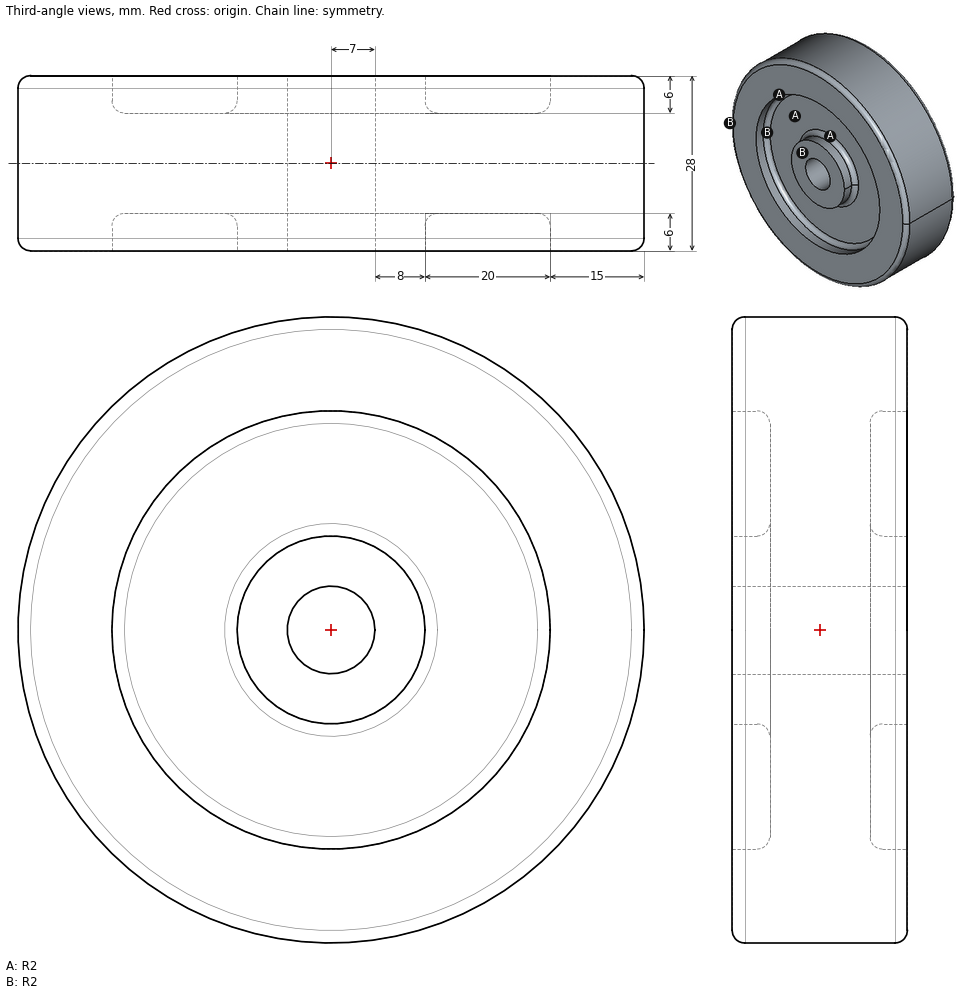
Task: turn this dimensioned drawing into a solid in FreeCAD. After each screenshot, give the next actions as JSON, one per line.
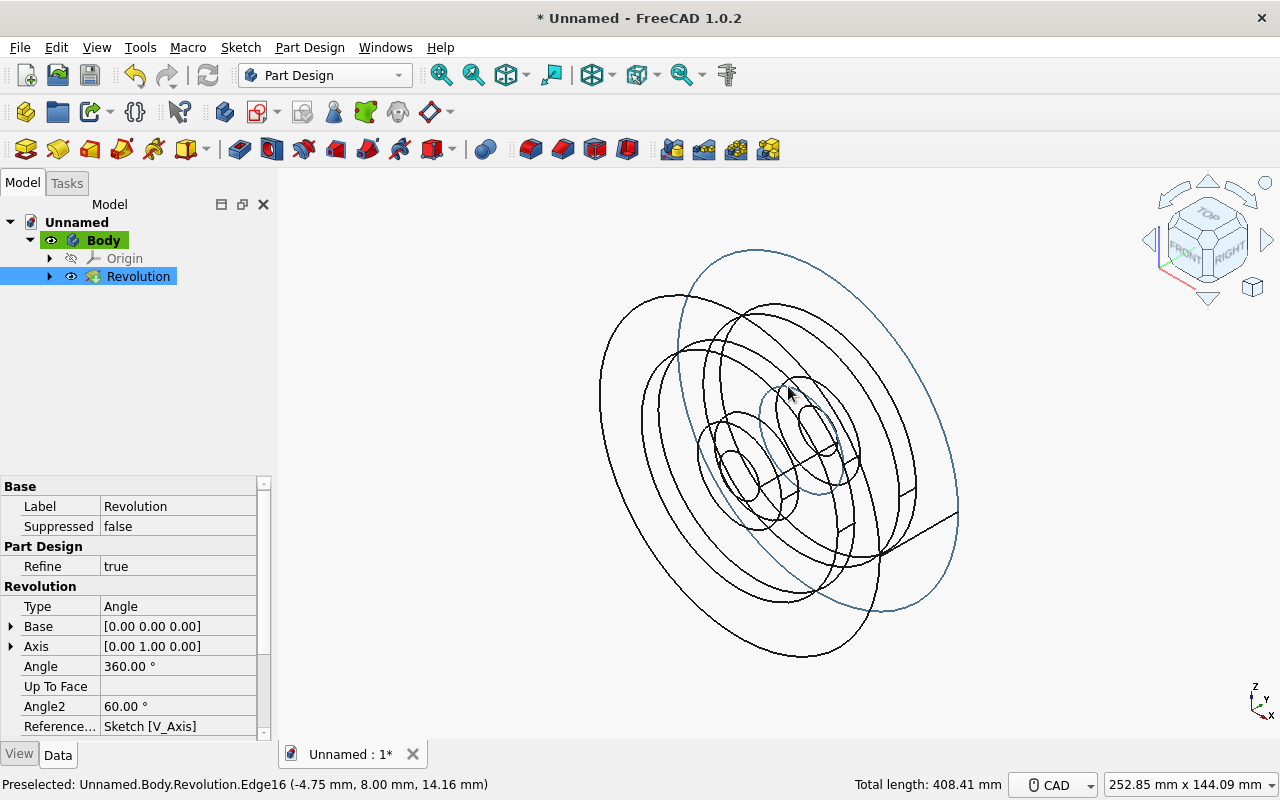
{"action": "left_click", "coordinate": [703, 383], "text": "ctrl"}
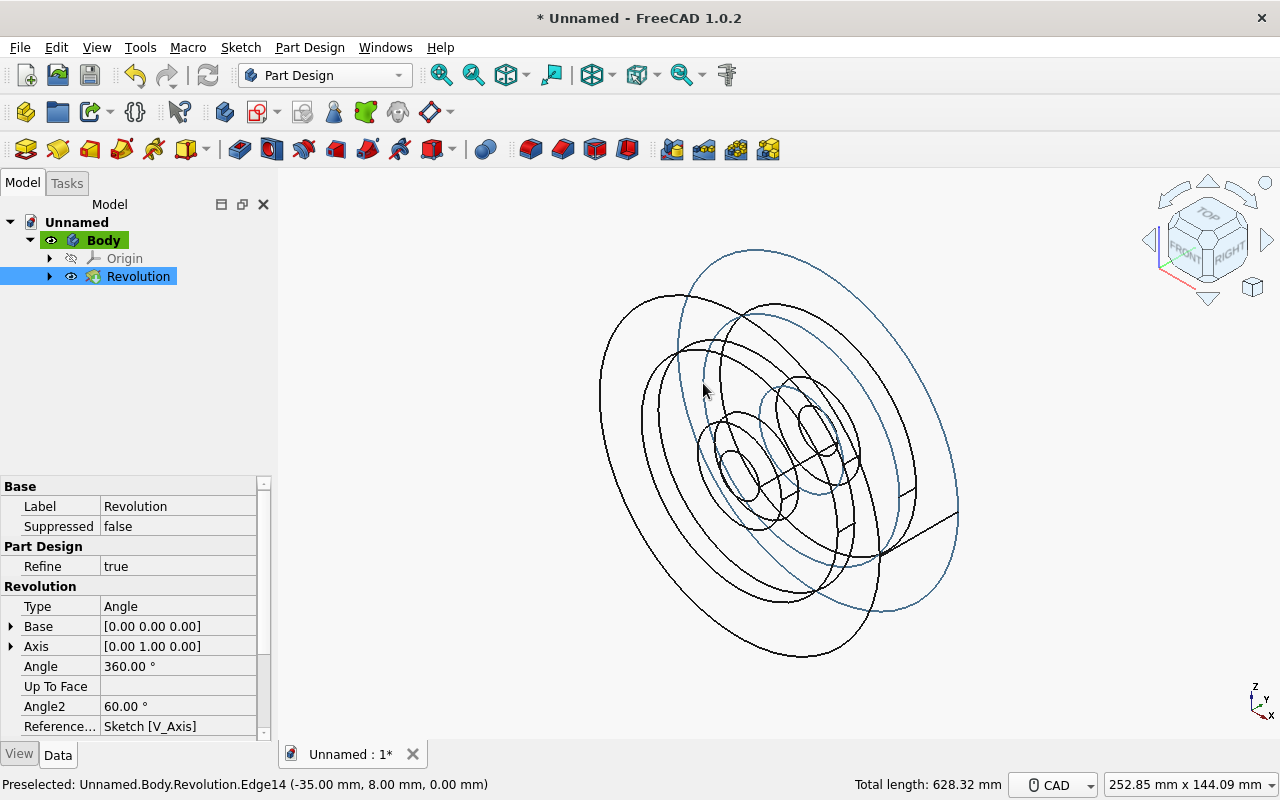
{"action": "key", "text": "v 1"}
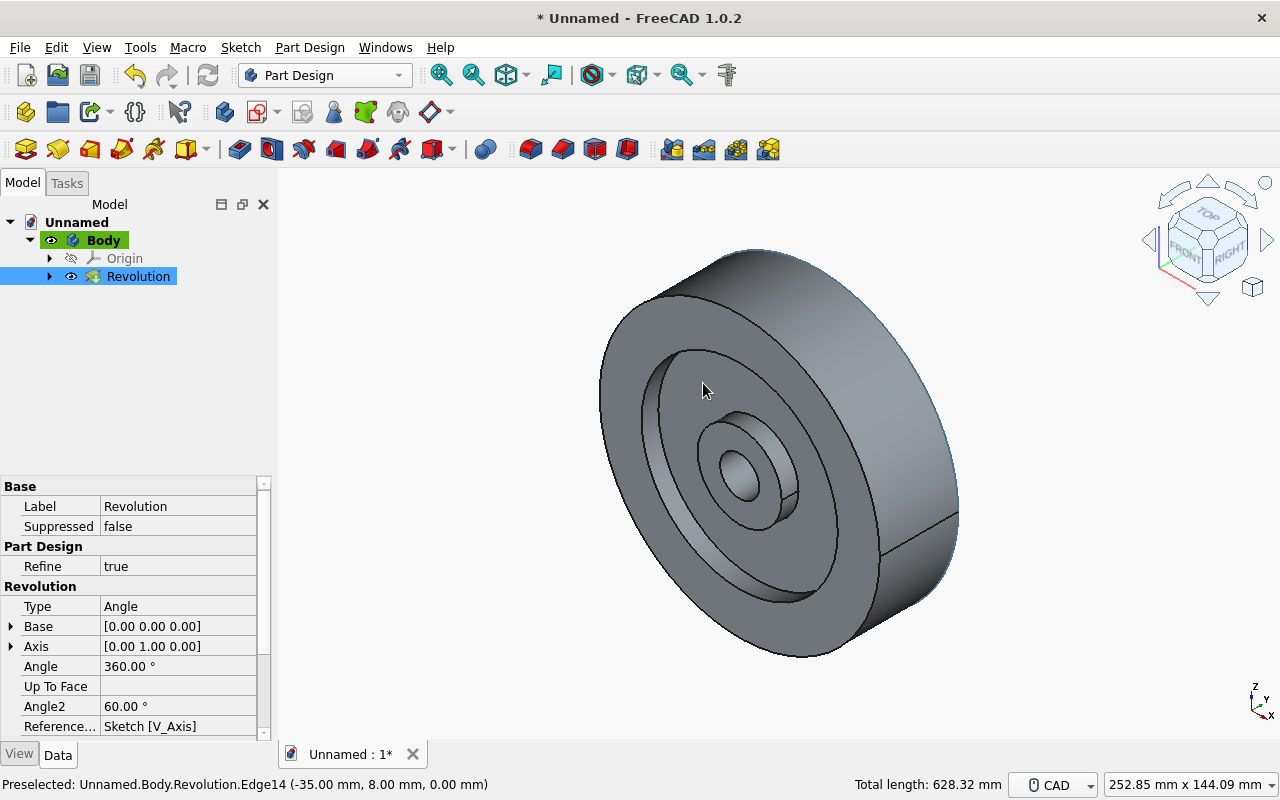
{"action": "left_click", "coordinate": [532, 150]}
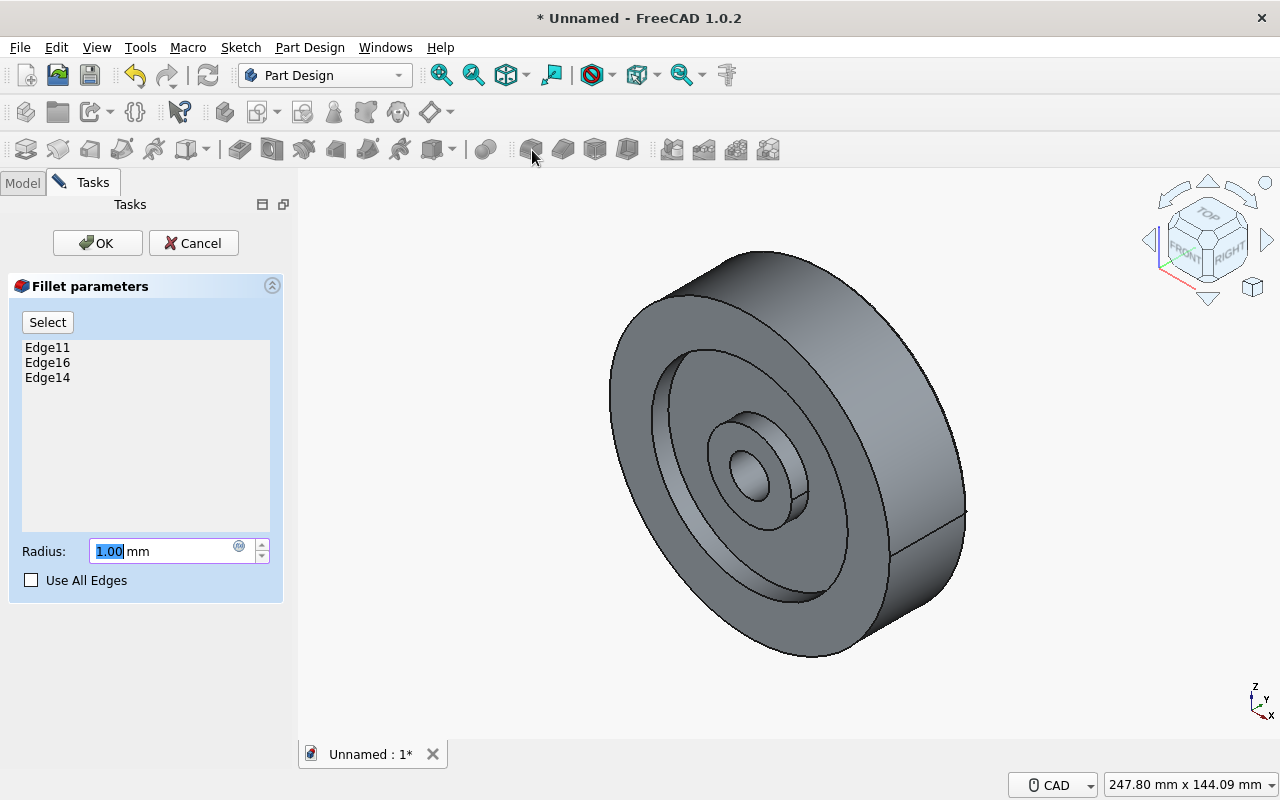
{"action": "type", "text": "2"}
{"action": "key", "text": "Tab"}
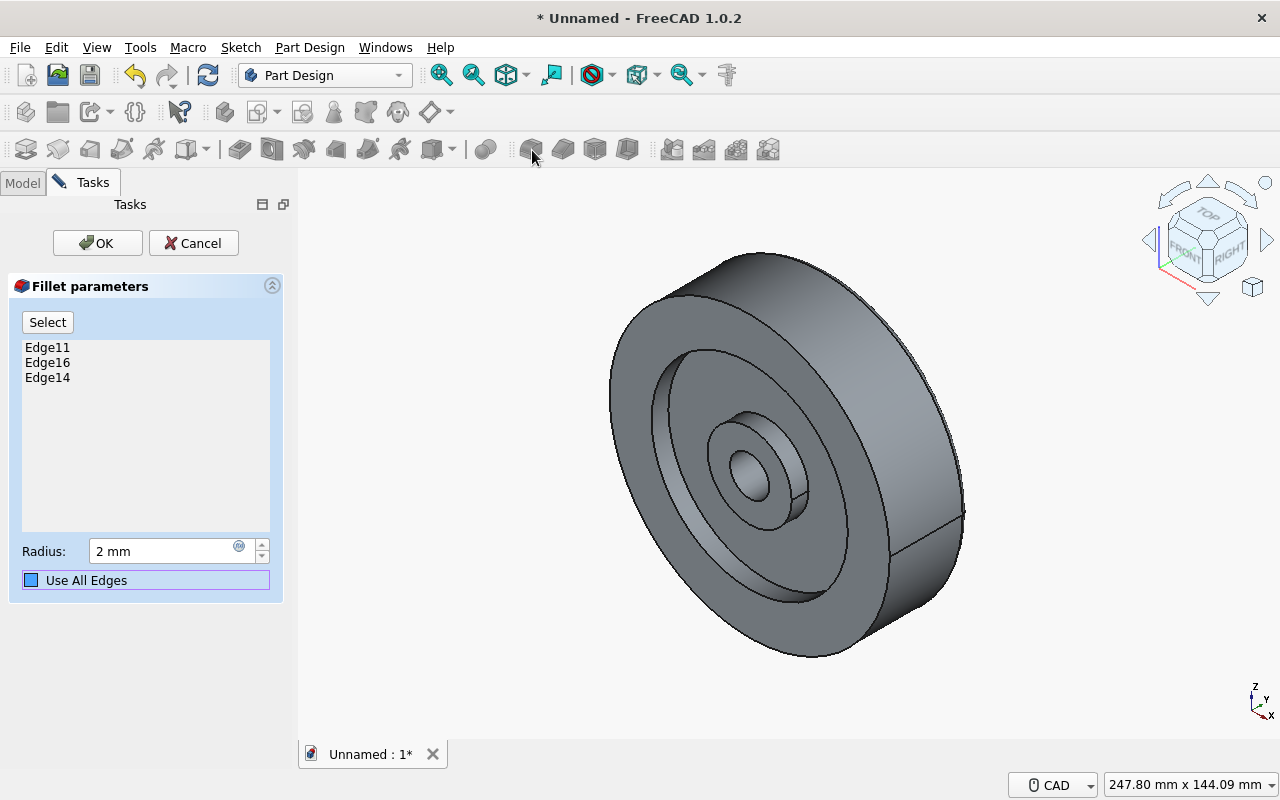
{"action": "left_click", "coordinate": [98, 243]}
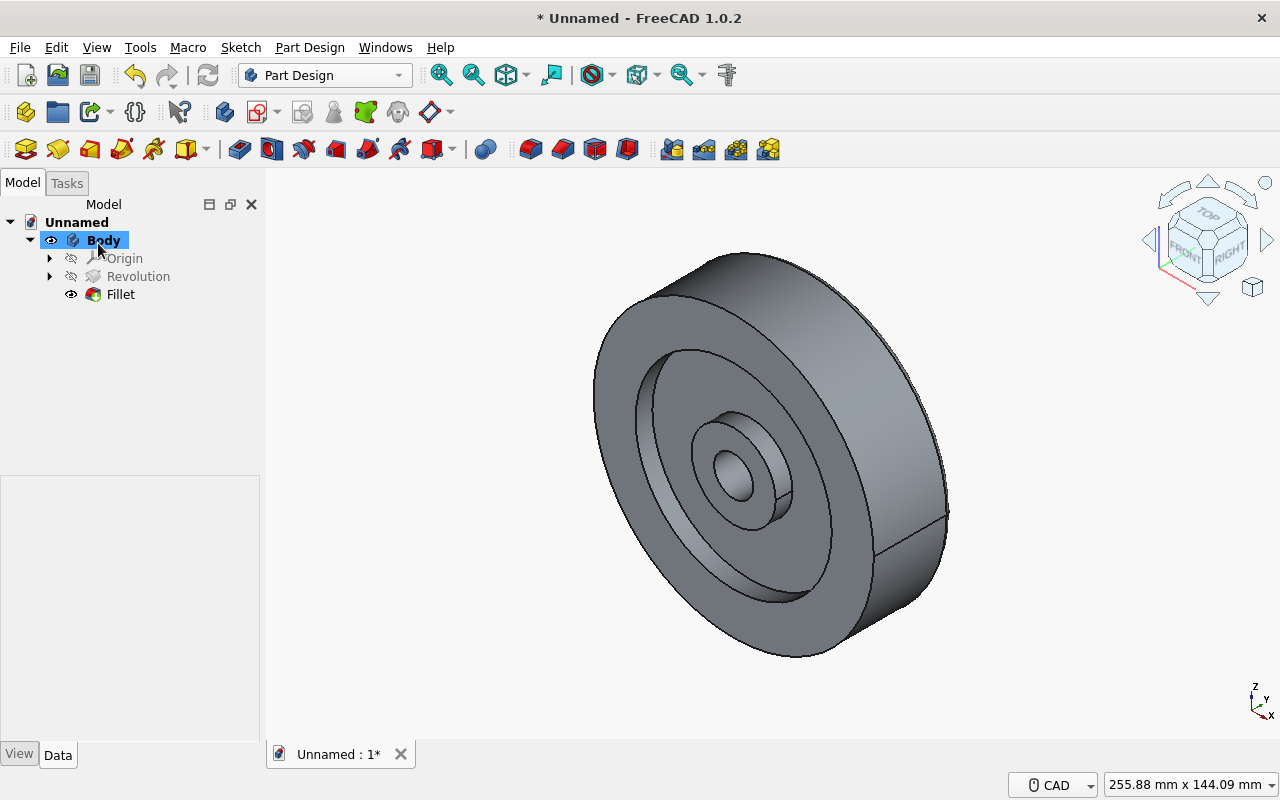
{"action": "left_click", "coordinate": [690, 296]}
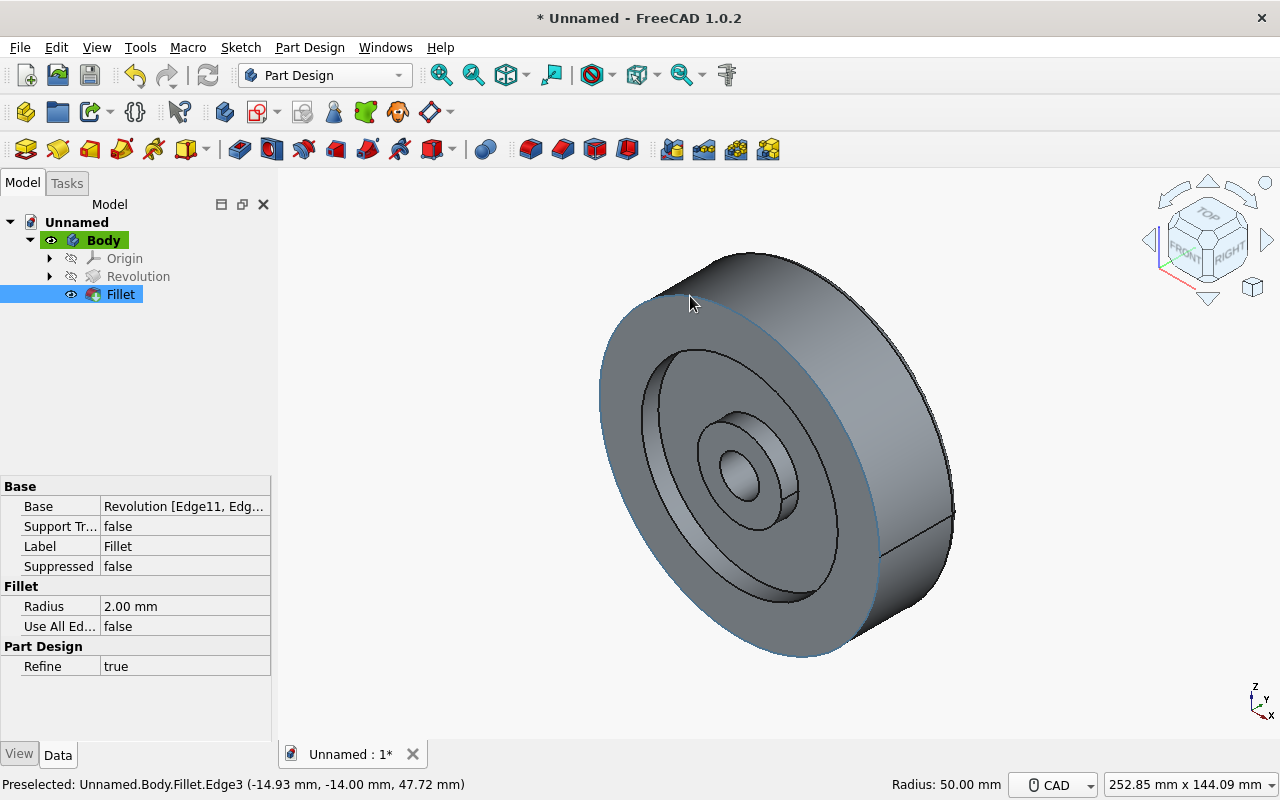
{"action": "key", "text": "2"}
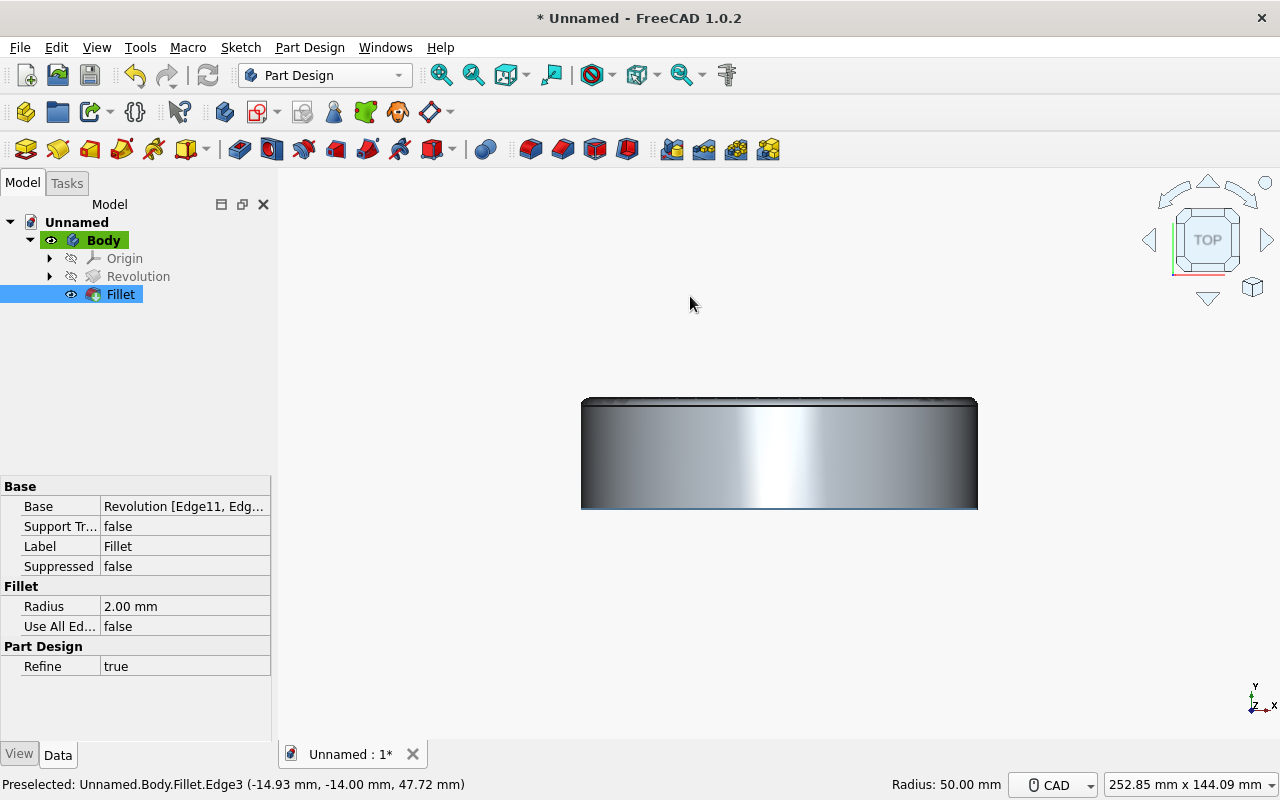
{"action": "left_click", "coordinate": [442, 76]}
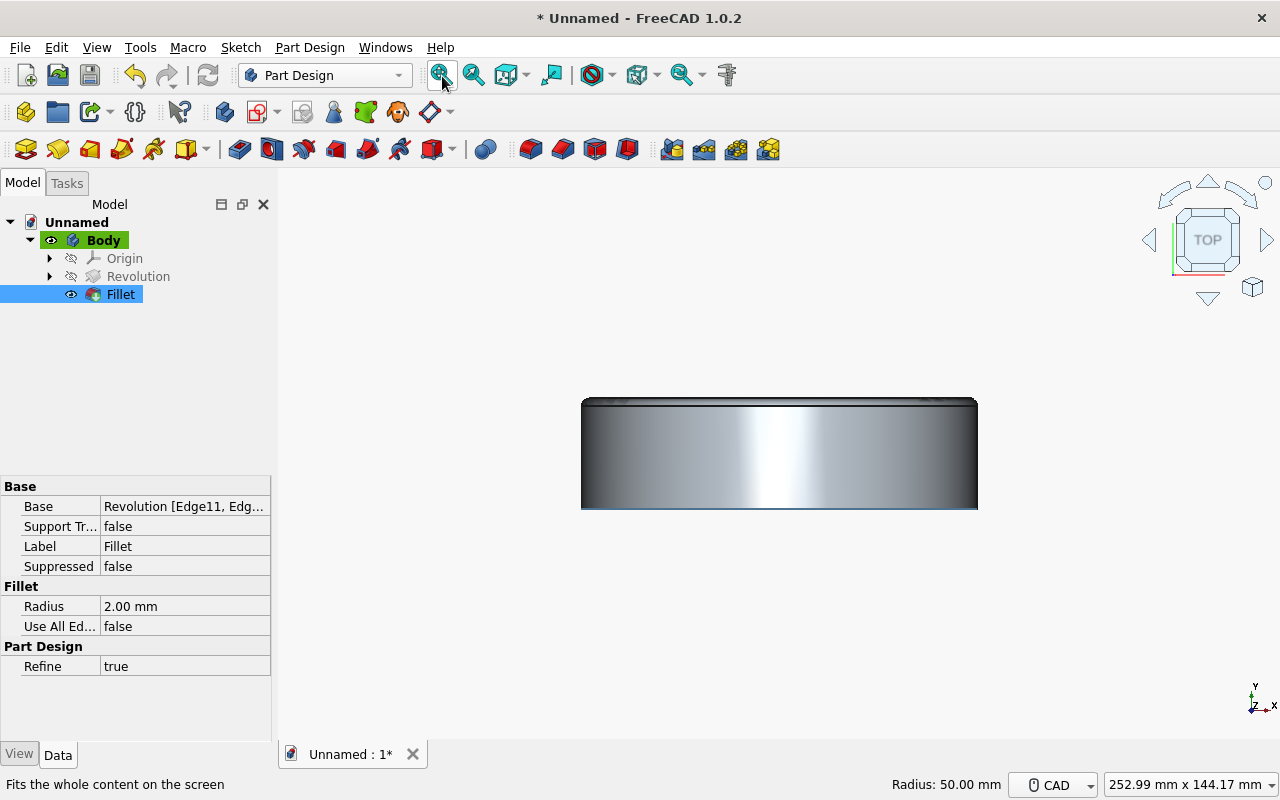
{"action": "key", "text": "0"}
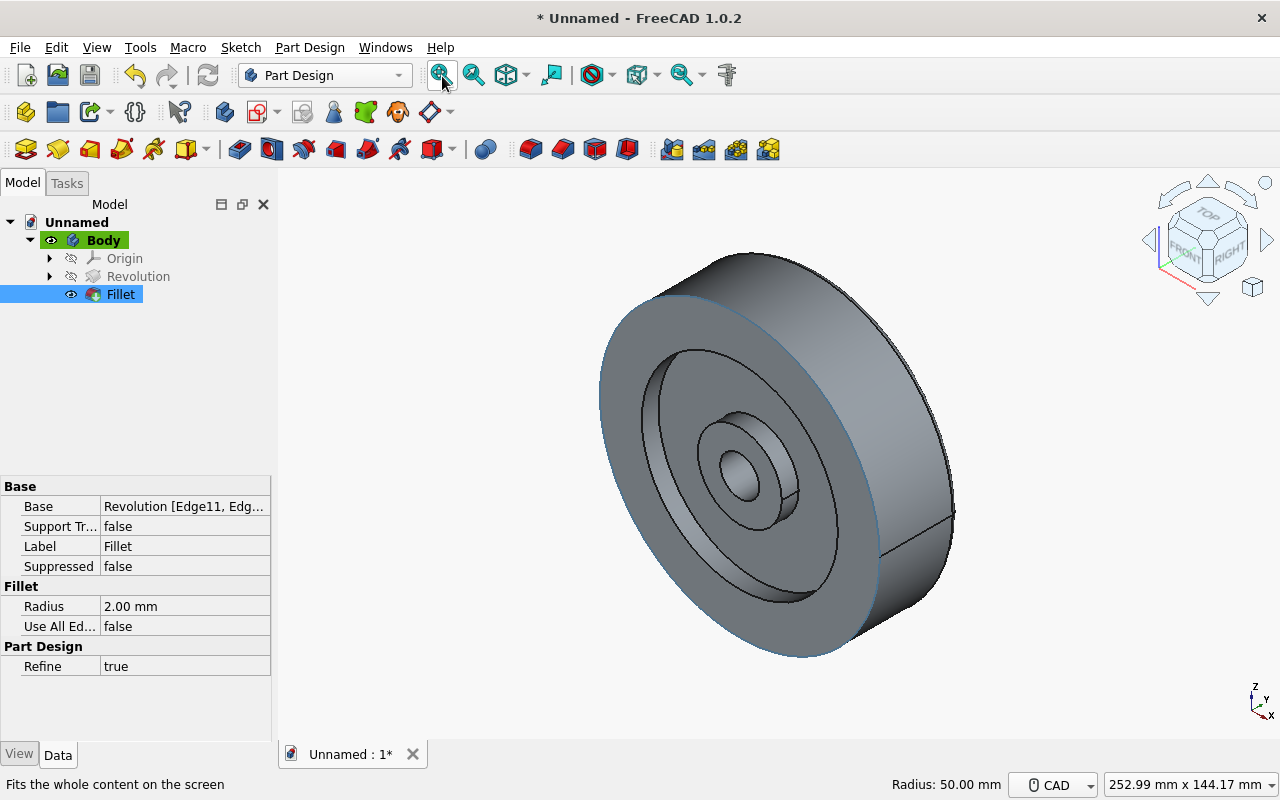
{"action": "key", "text": "1"}